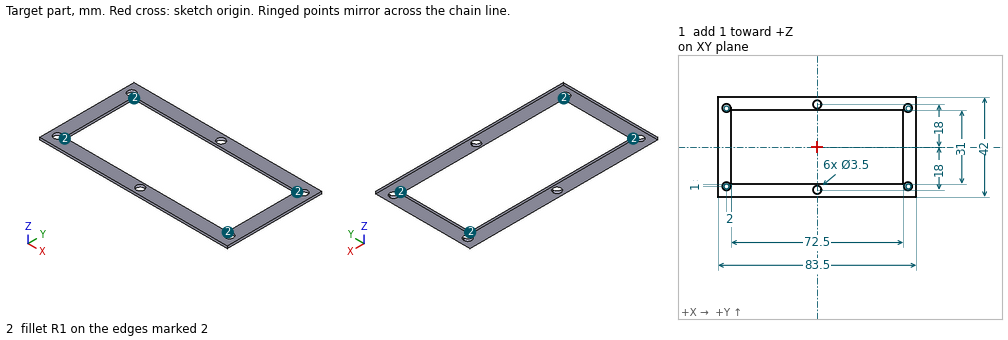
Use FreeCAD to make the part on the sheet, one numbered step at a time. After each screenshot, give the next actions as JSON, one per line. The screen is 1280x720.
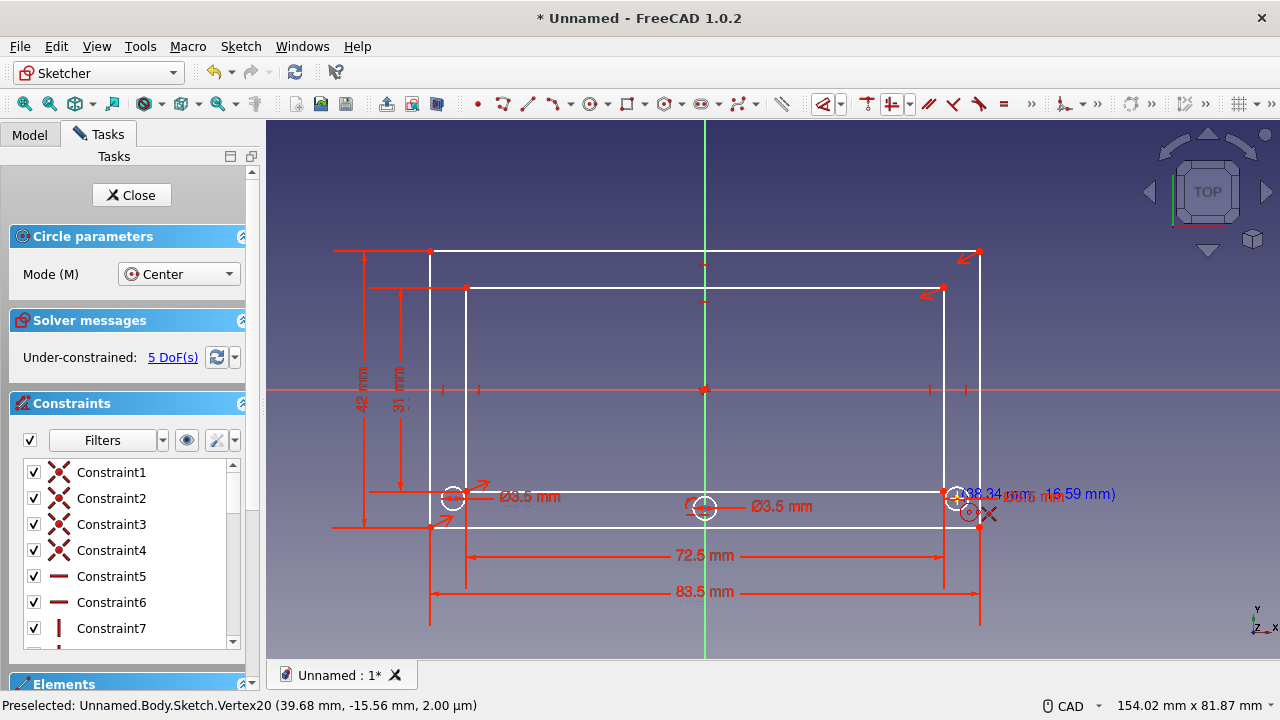
{"action": "scroll", "coordinate": [453, 281], "scroll_direction": "up", "scroll_amount": 4}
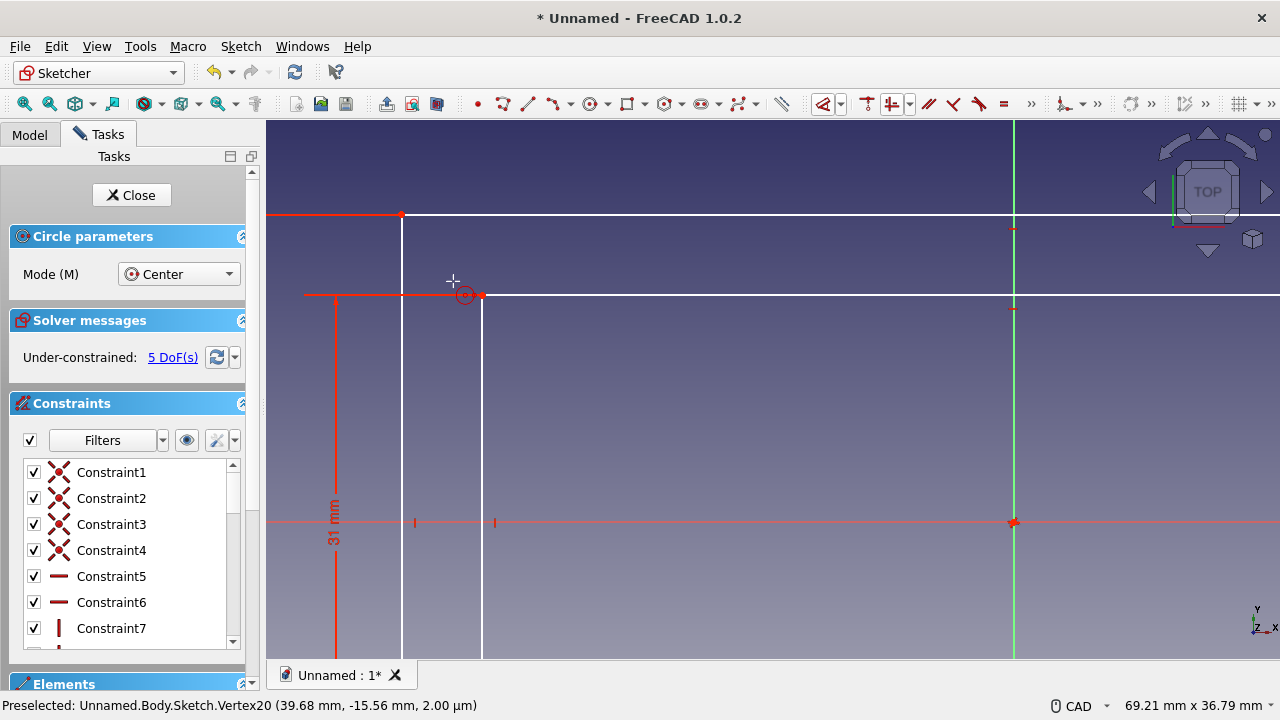
{"action": "left_click", "coordinate": [453, 281]}
{"action": "mouse_move", "coordinate": [471, 262]}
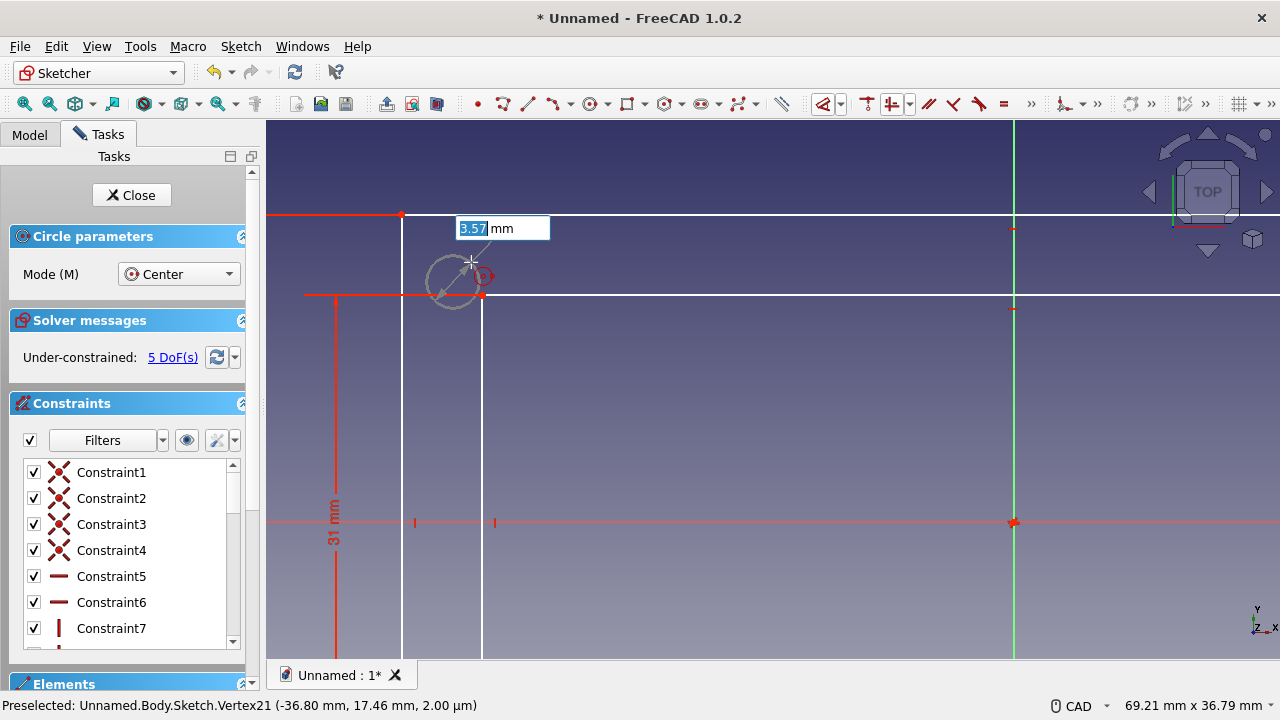
{"action": "type", "text": "3.5"}
{"action": "key", "text": "Return"}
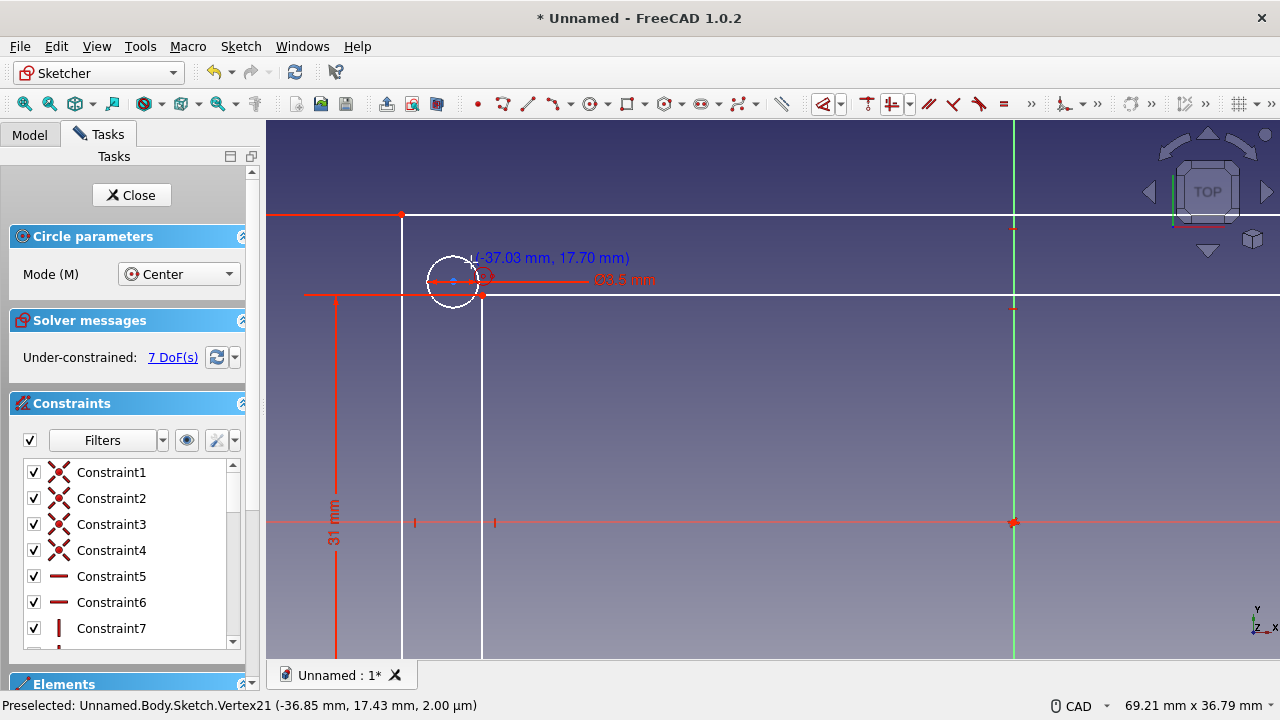
{"action": "left_click", "coordinate": [1014, 259]}
{"action": "mouse_move", "coordinate": [1032, 241]}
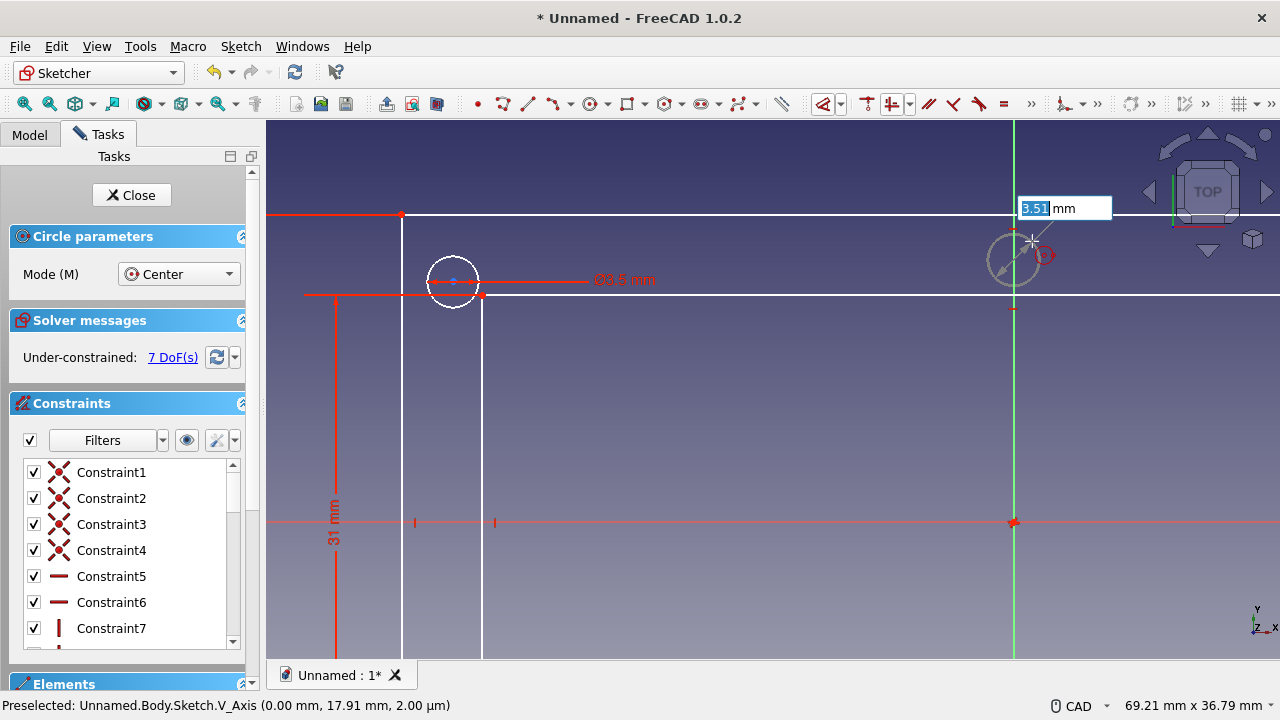
{"action": "type", "text": "3.5"}
{"action": "key", "text": "Return"}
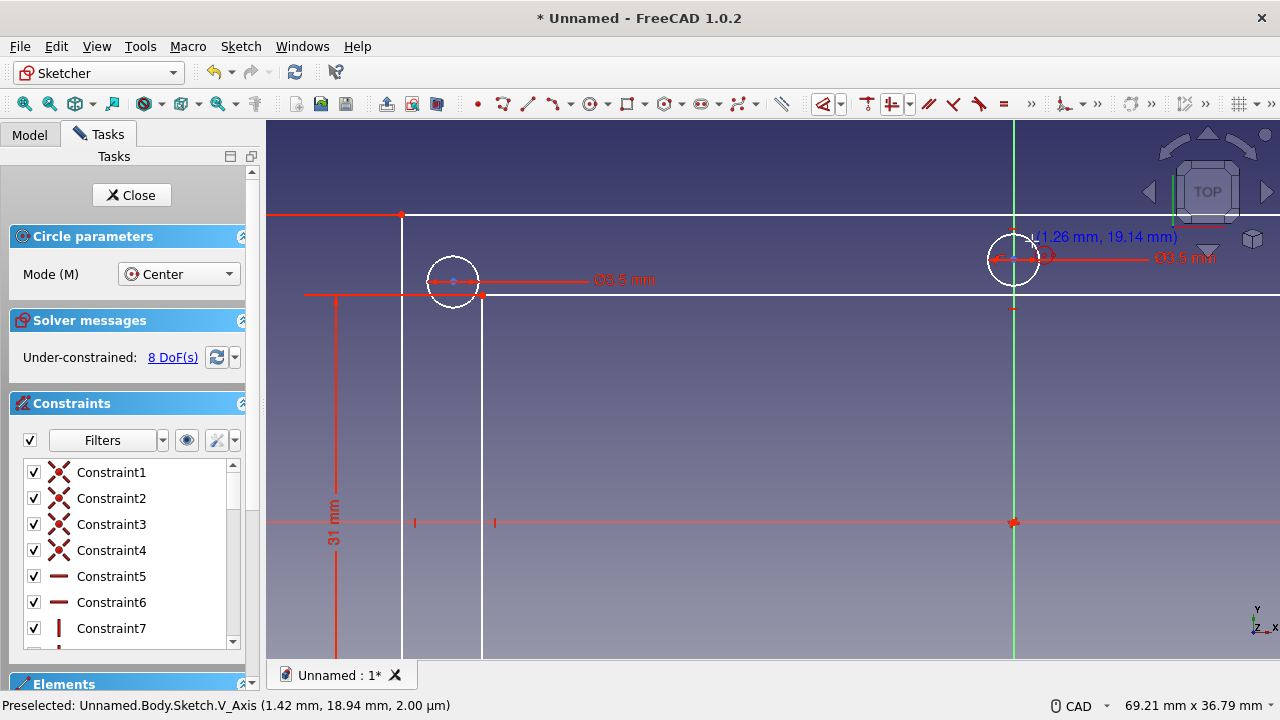
{"action": "scroll", "coordinate": [452, 281], "scroll_direction": "down", "scroll_amount": 4}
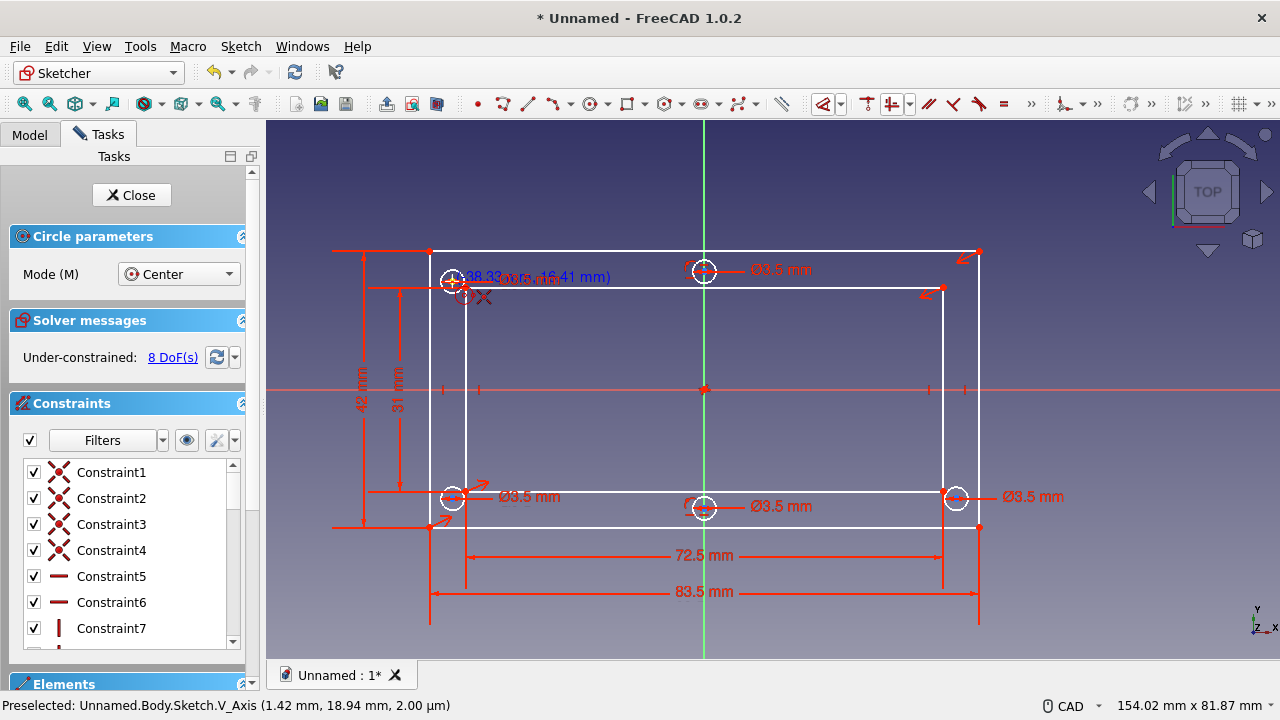
{"action": "scroll", "coordinate": [956, 281], "scroll_direction": "up", "scroll_amount": 4}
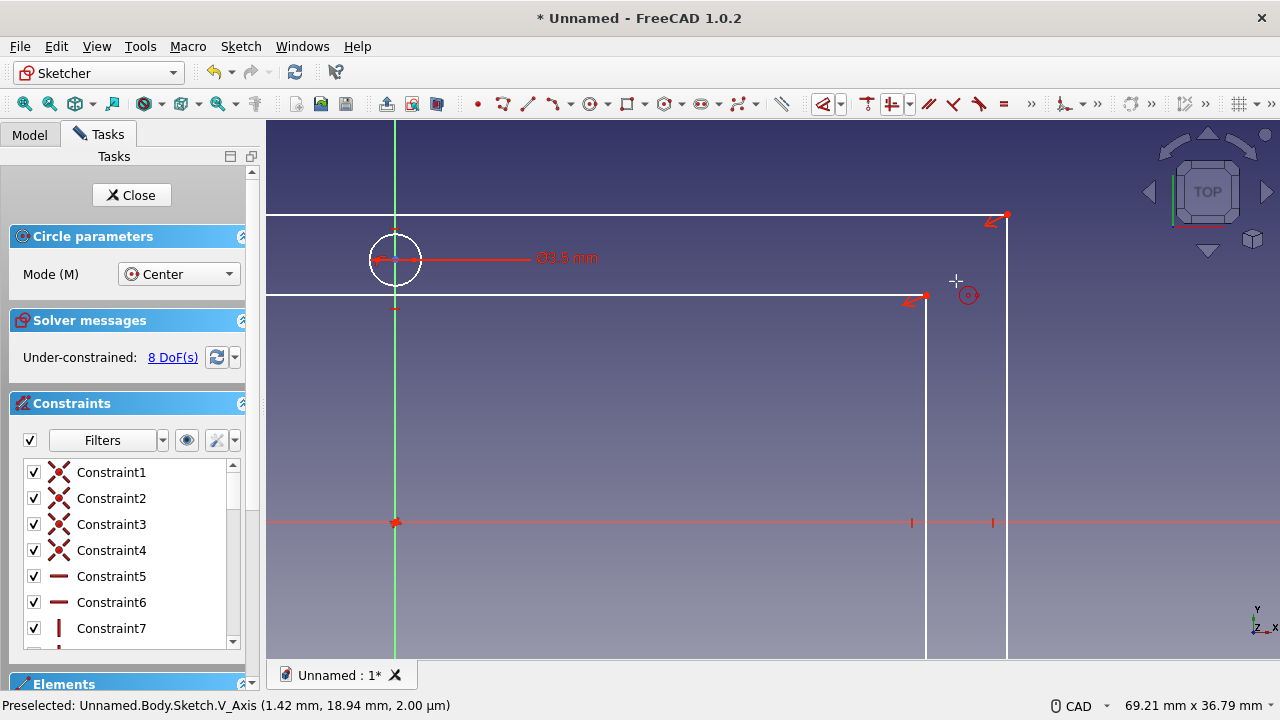
{"action": "left_click", "coordinate": [956, 281]}
{"action": "mouse_move", "coordinate": [974, 262]}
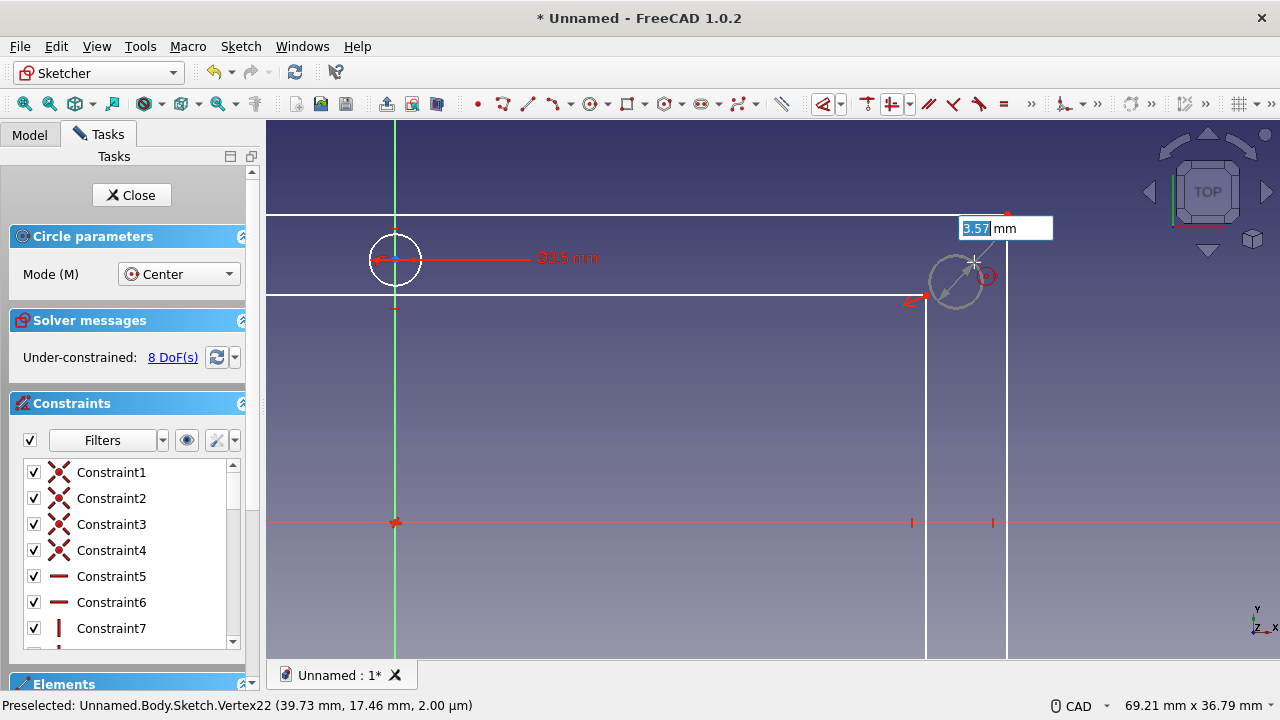
{"action": "type", "text": "3.5"}
{"action": "key", "text": "Return"}
{"action": "key", "text": "Escape"}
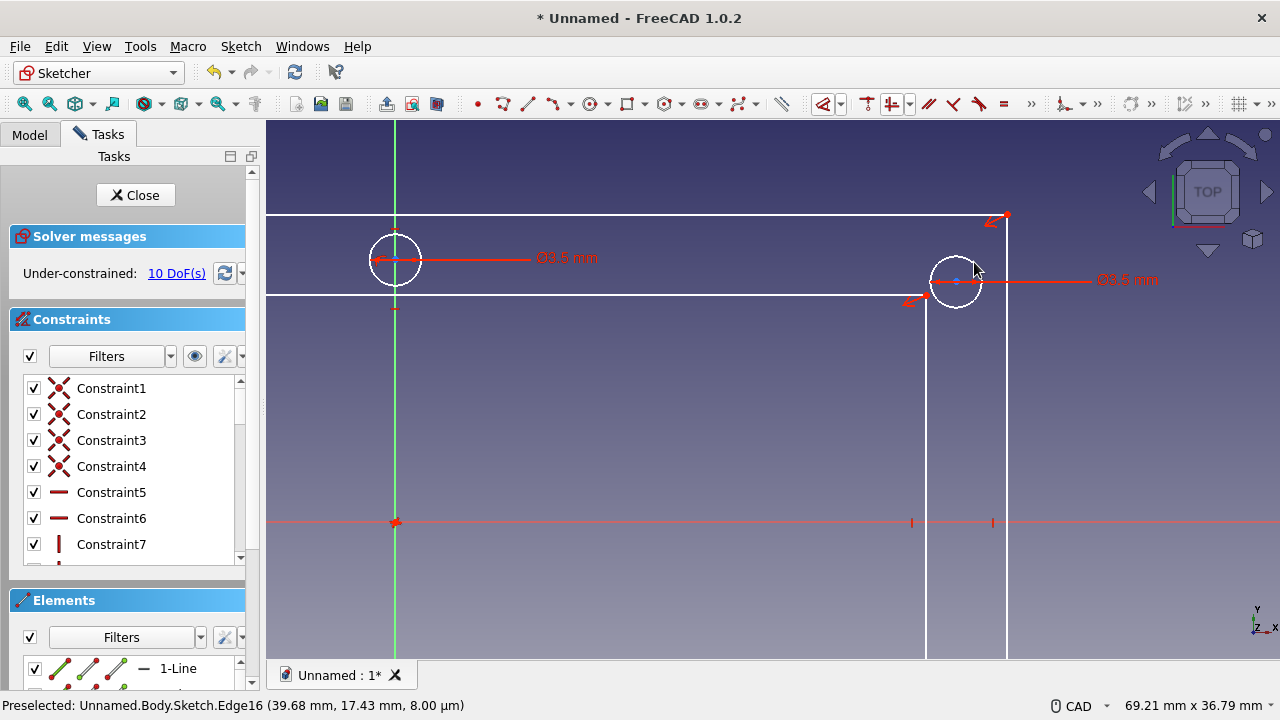
{"action": "scroll", "coordinate": [957, 281], "scroll_direction": "down", "scroll_amount": 4}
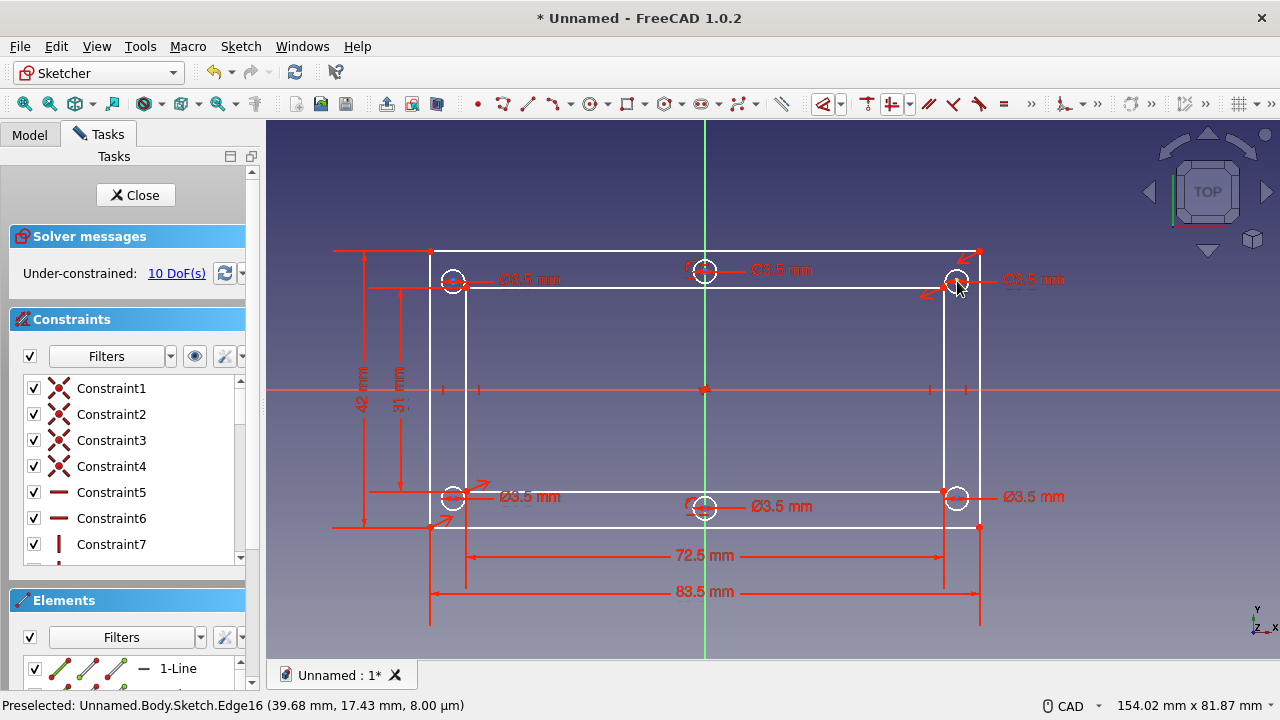
{"action": "left_click", "coordinate": [453, 499]}